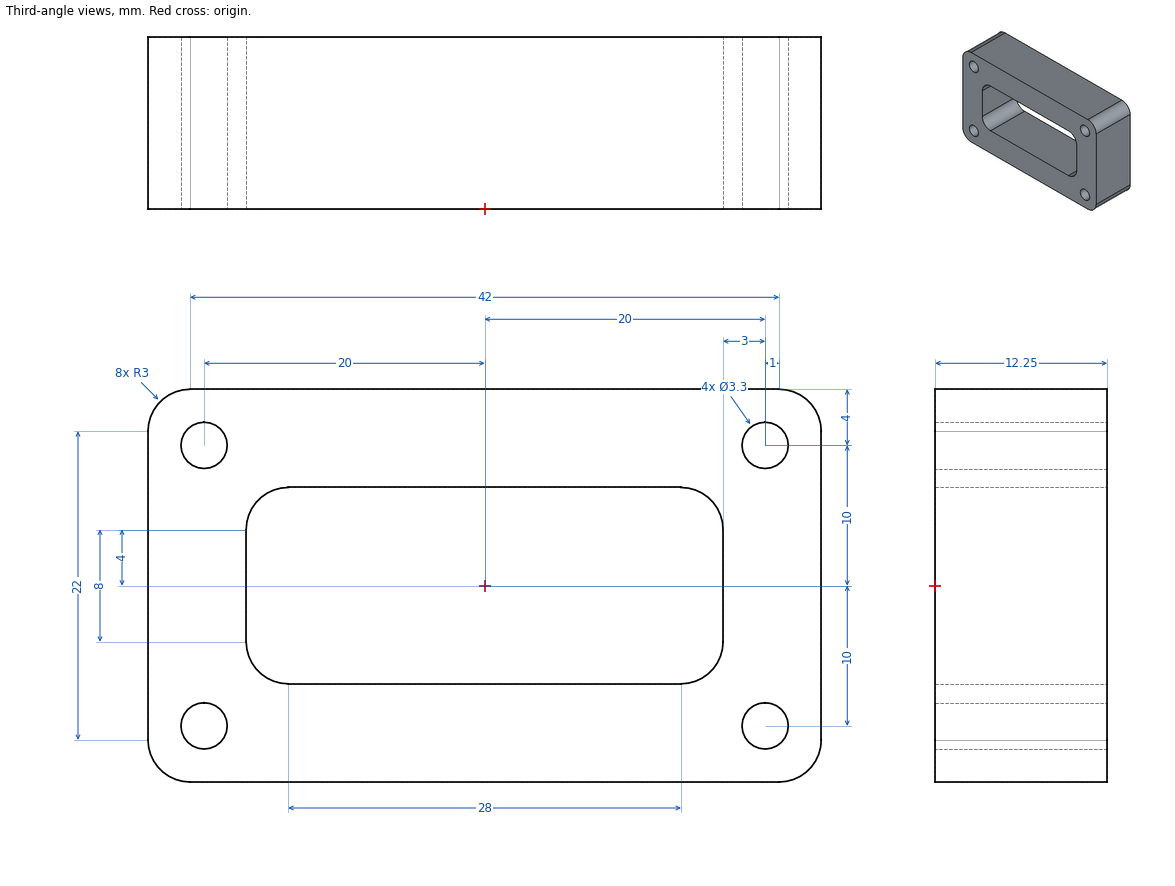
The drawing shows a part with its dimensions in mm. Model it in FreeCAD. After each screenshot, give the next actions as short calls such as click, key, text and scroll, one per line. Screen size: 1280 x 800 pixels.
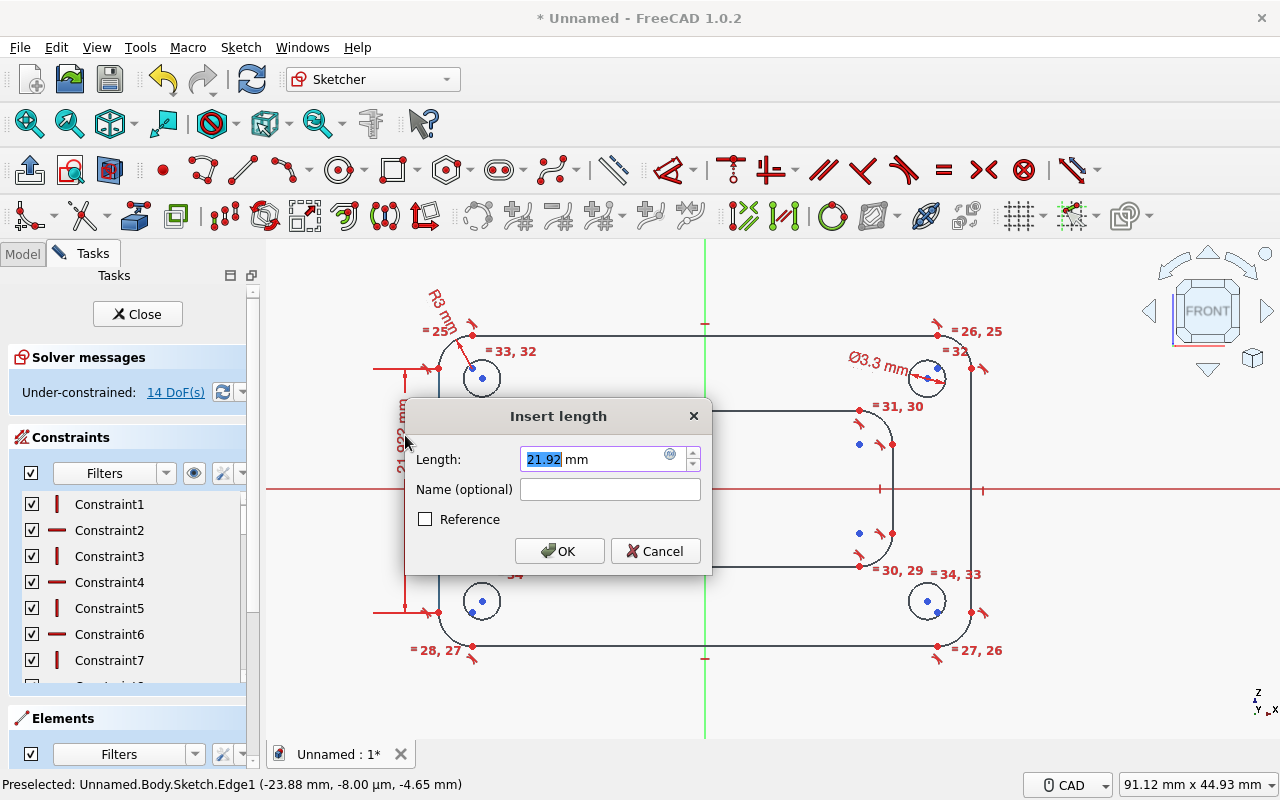
text(22)
key(Return)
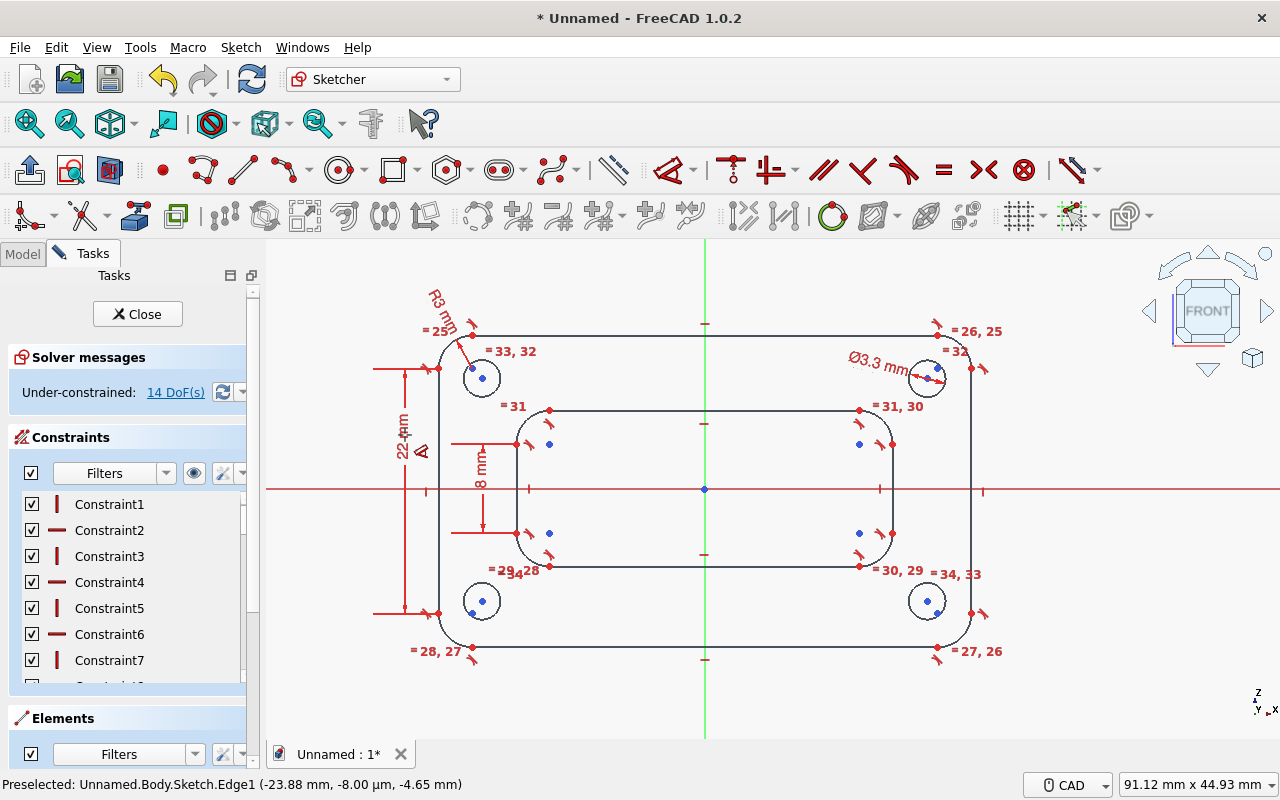
click(612, 336)
click(598, 302)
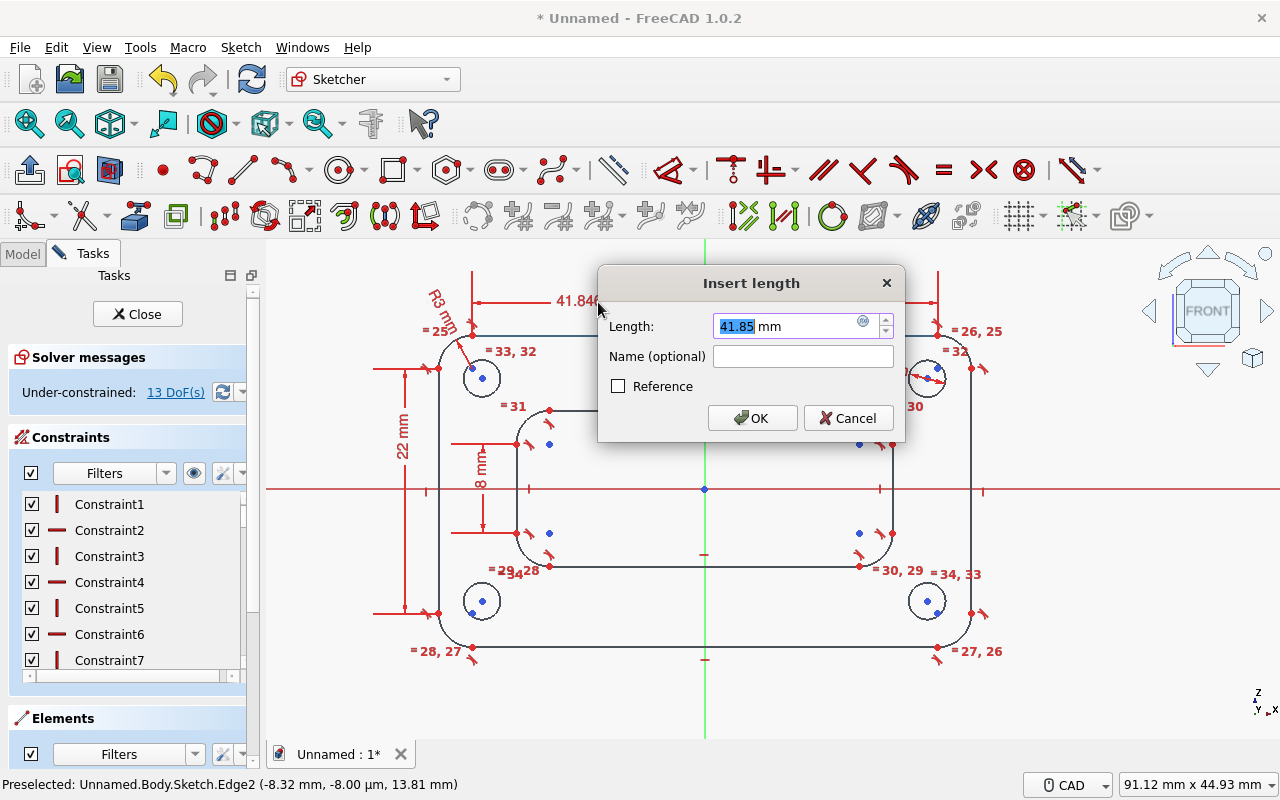
text(42)
key(Return)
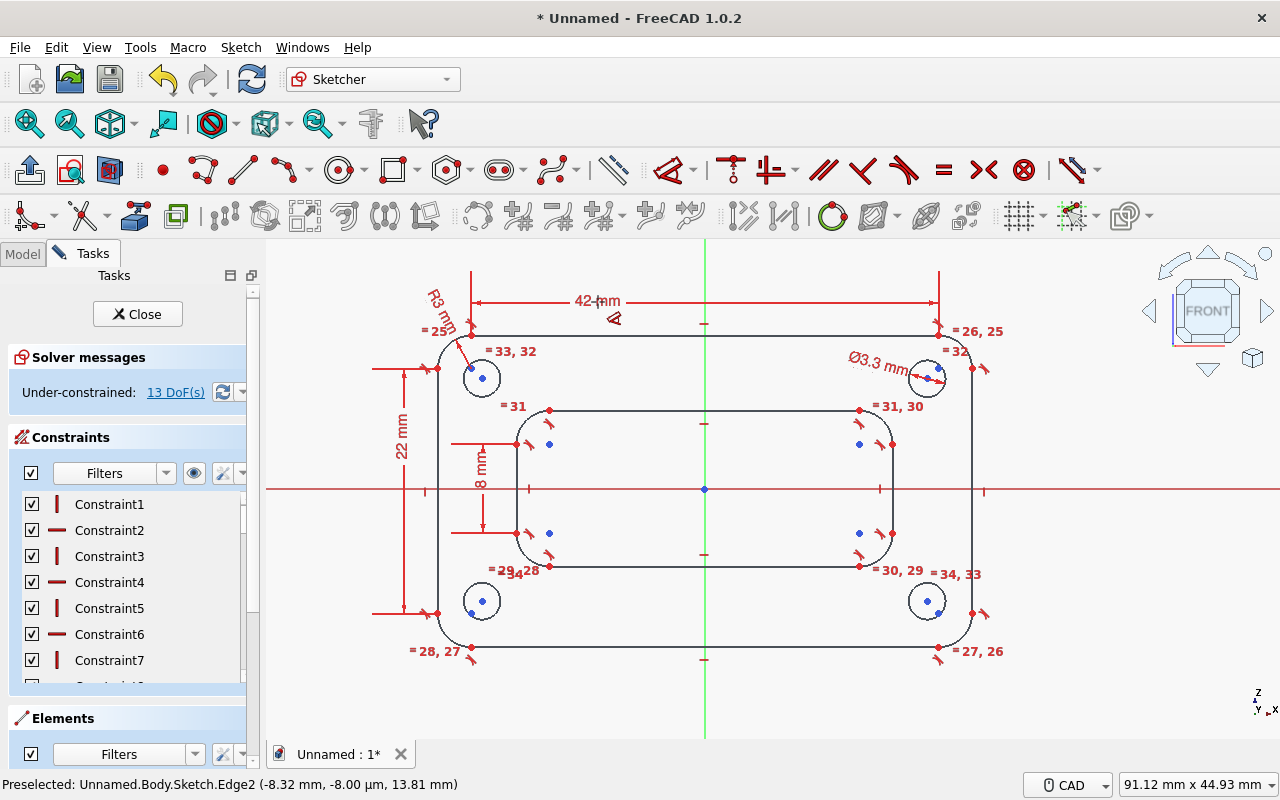
click(643, 567)
click(633, 601)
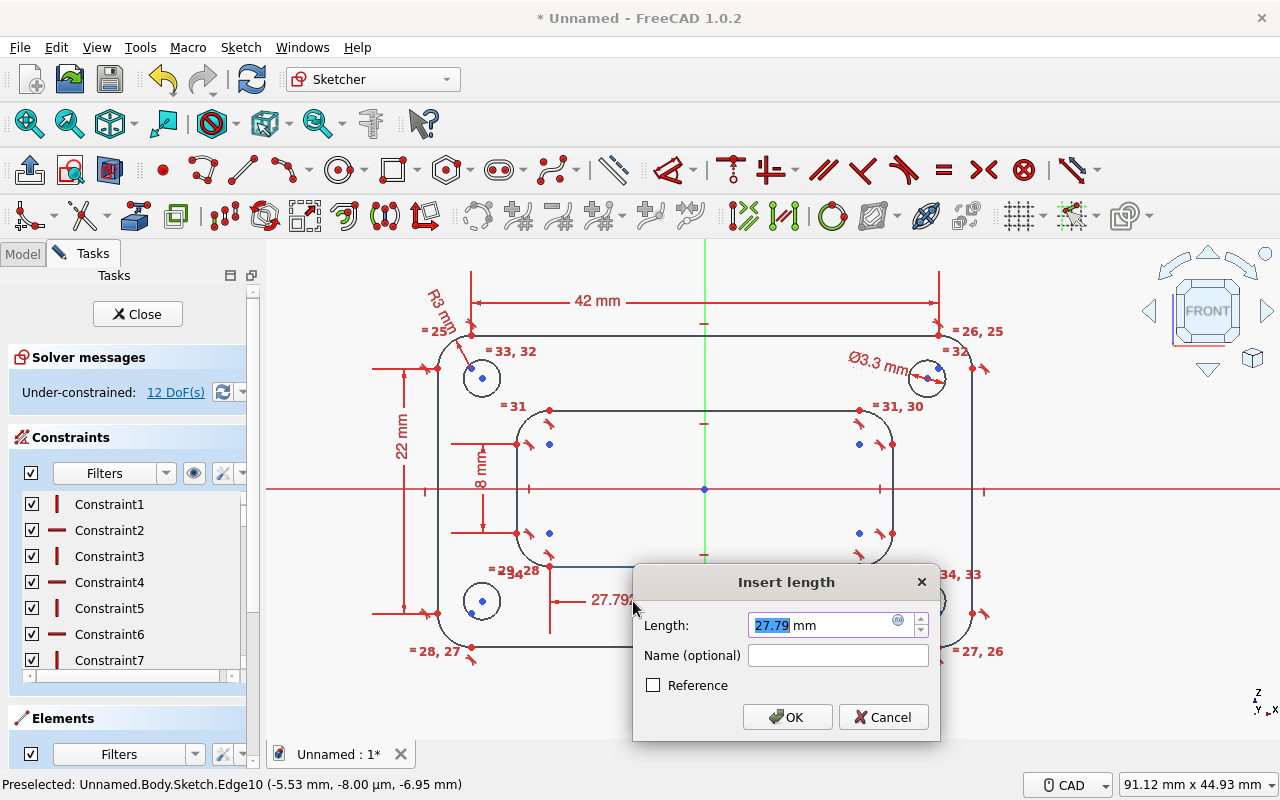
text(28)
key(Return)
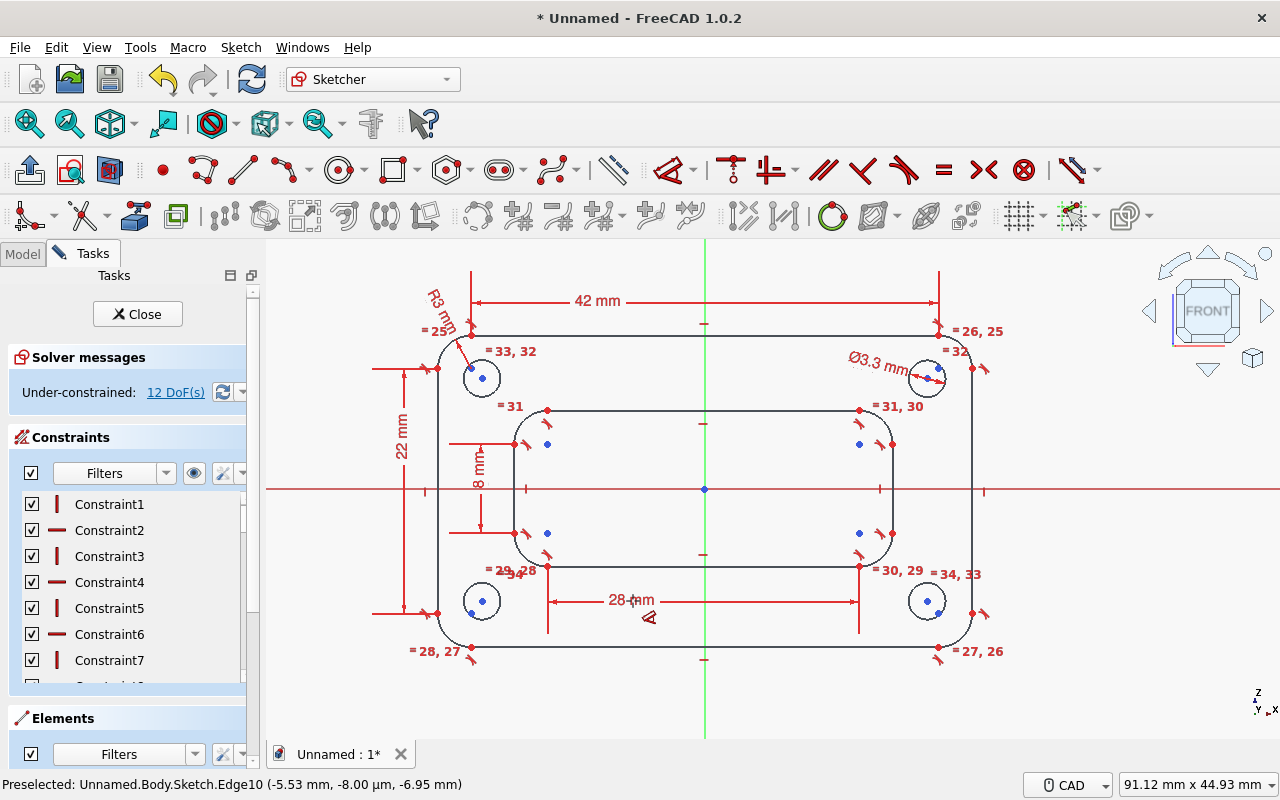
click(514, 444)
click(739, 467)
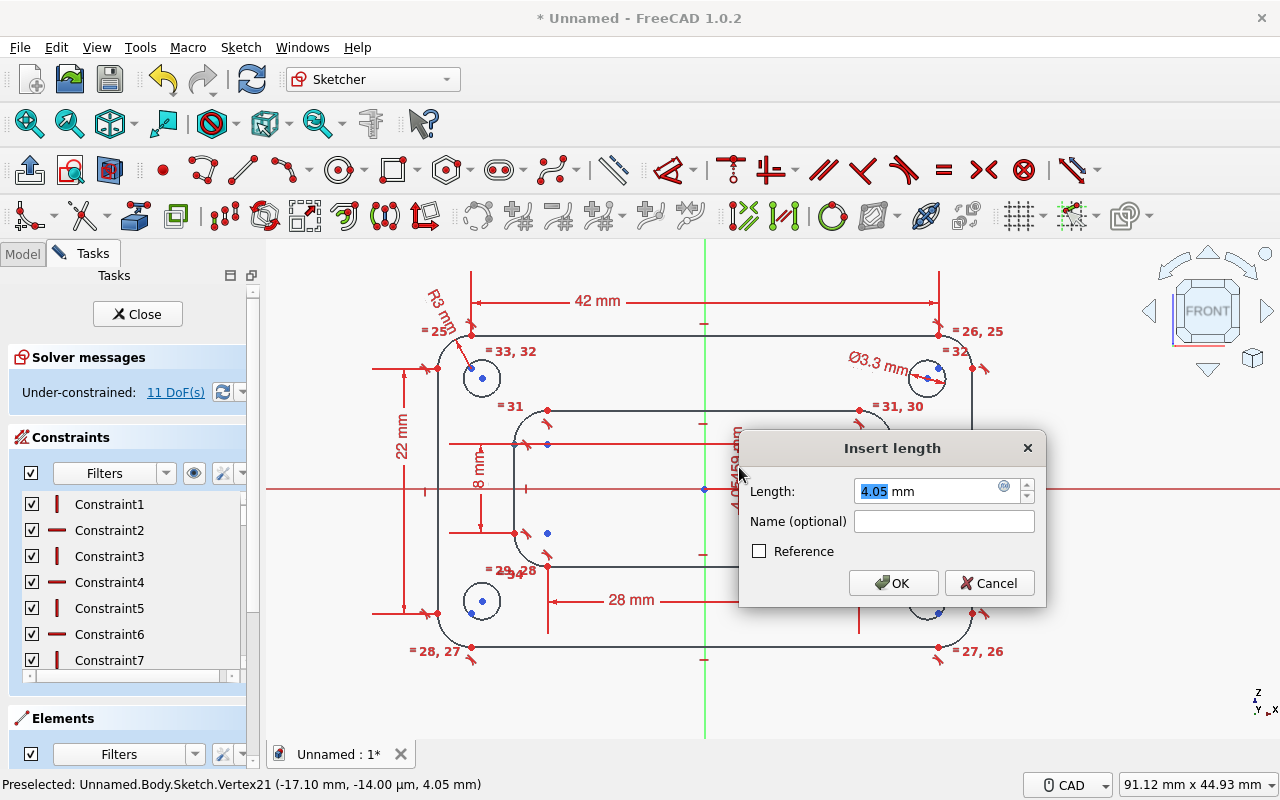
text(4)
key(Return)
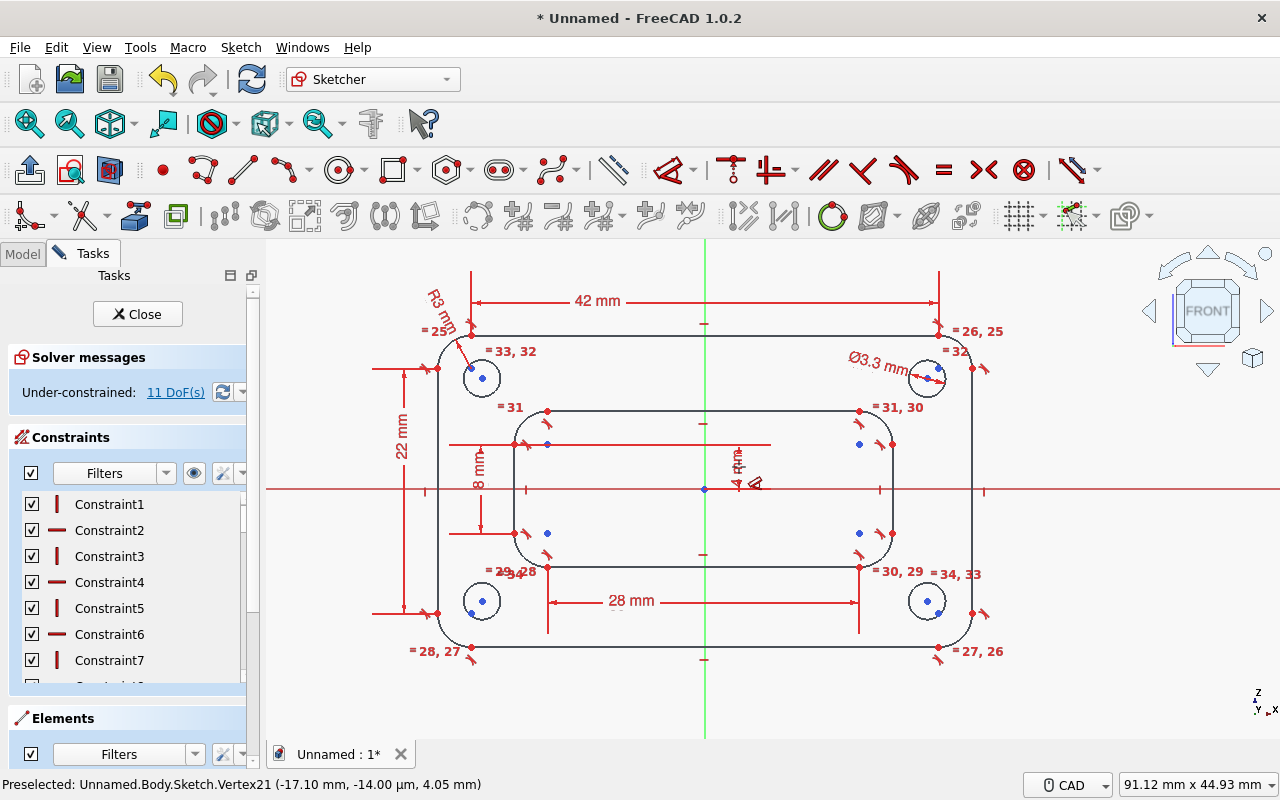
click(927, 379)
click(816, 523)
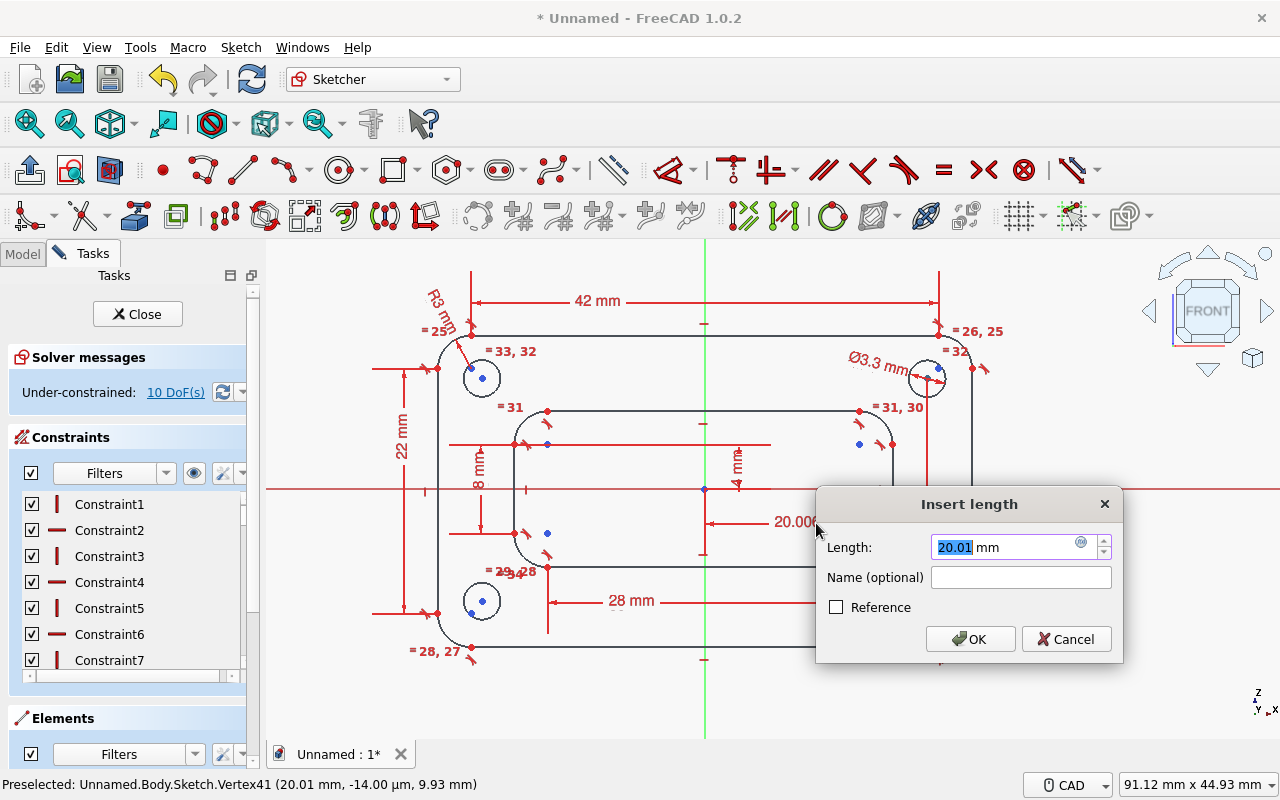
text(20)
key(Return)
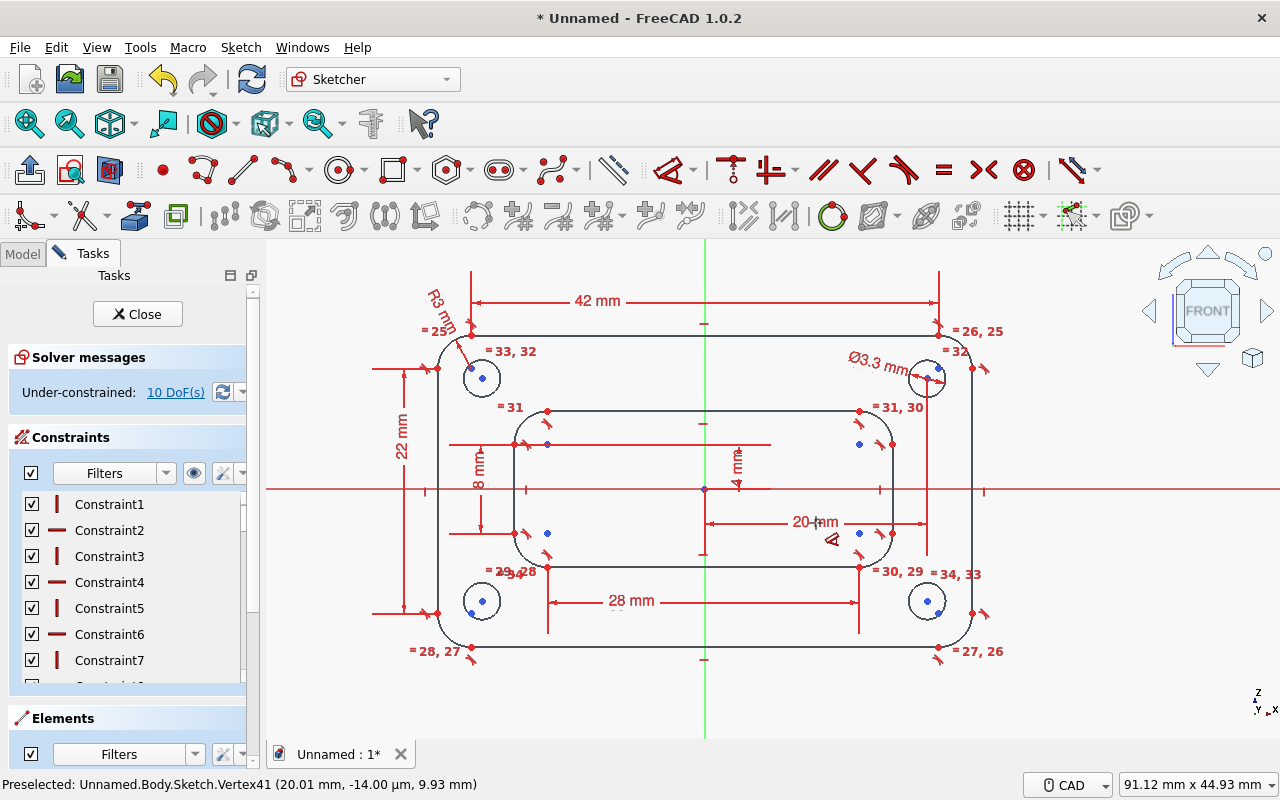
click(927, 379)
click(671, 434)